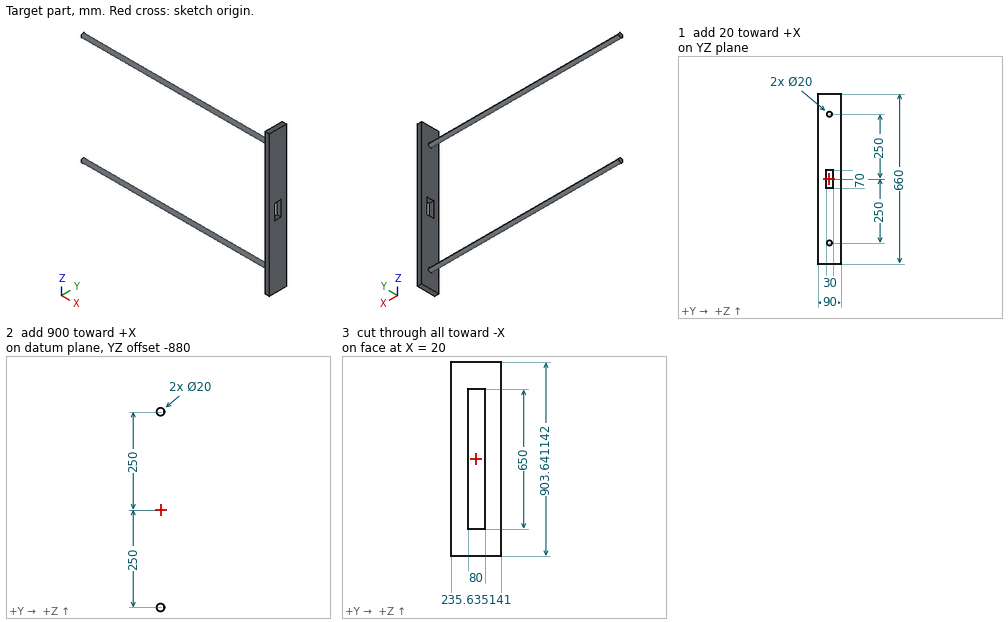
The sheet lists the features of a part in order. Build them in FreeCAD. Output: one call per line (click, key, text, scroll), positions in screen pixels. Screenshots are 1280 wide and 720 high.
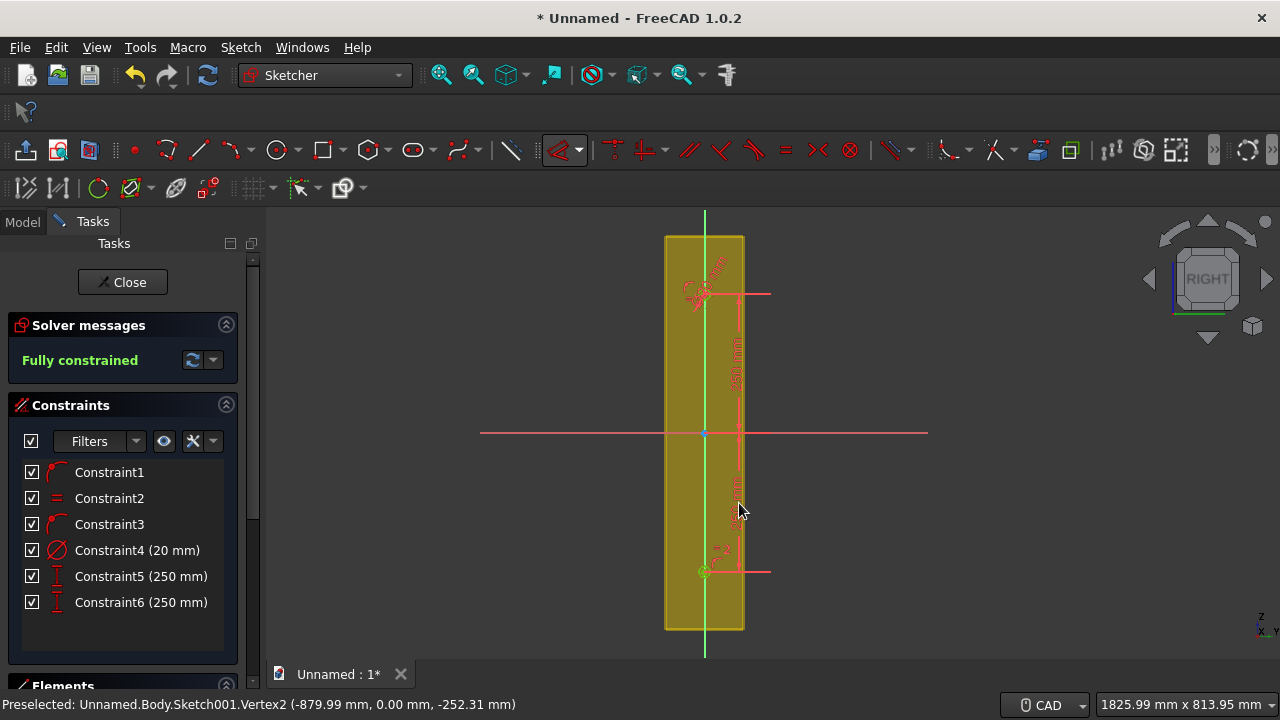
click(123, 282)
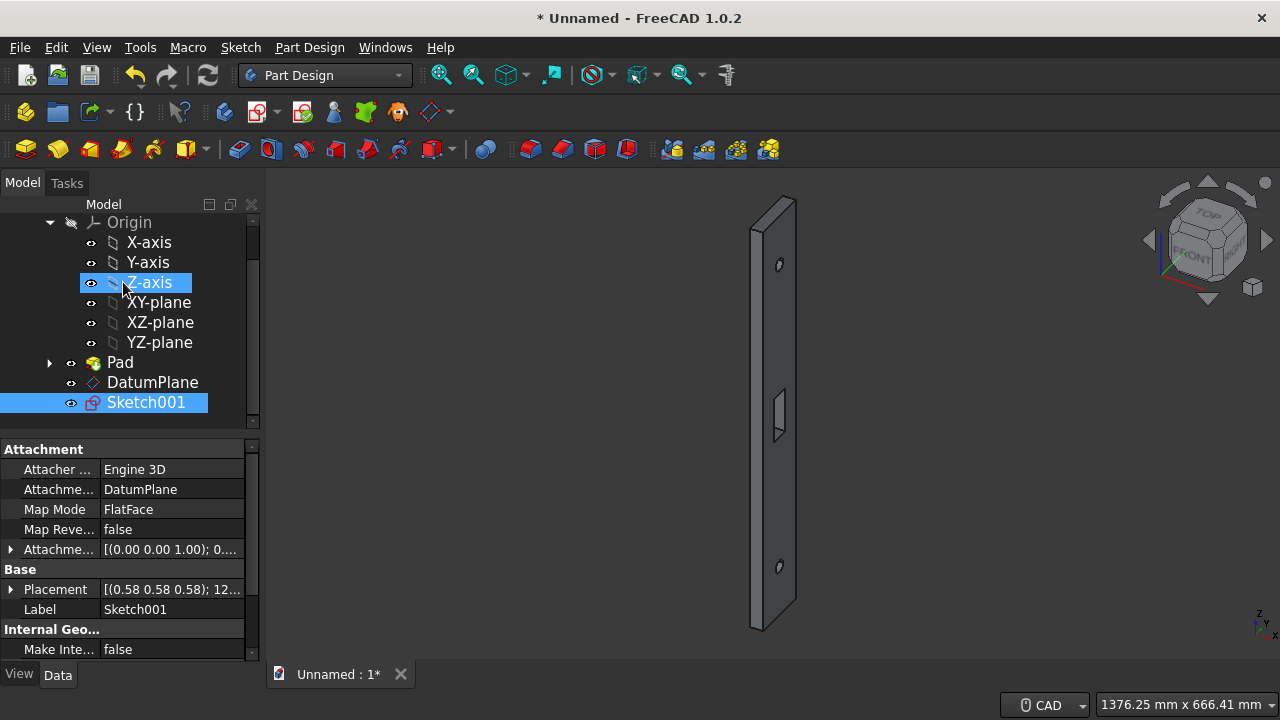
click(26, 150)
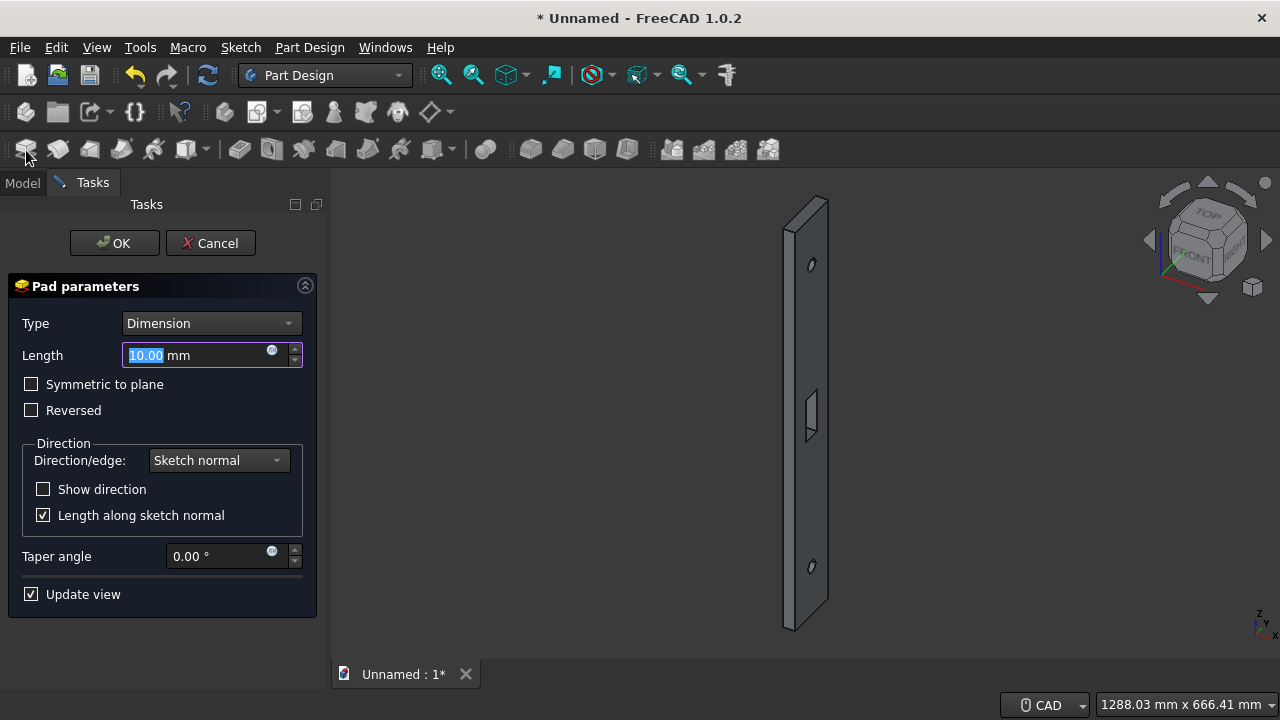
text(900)
key(Tab)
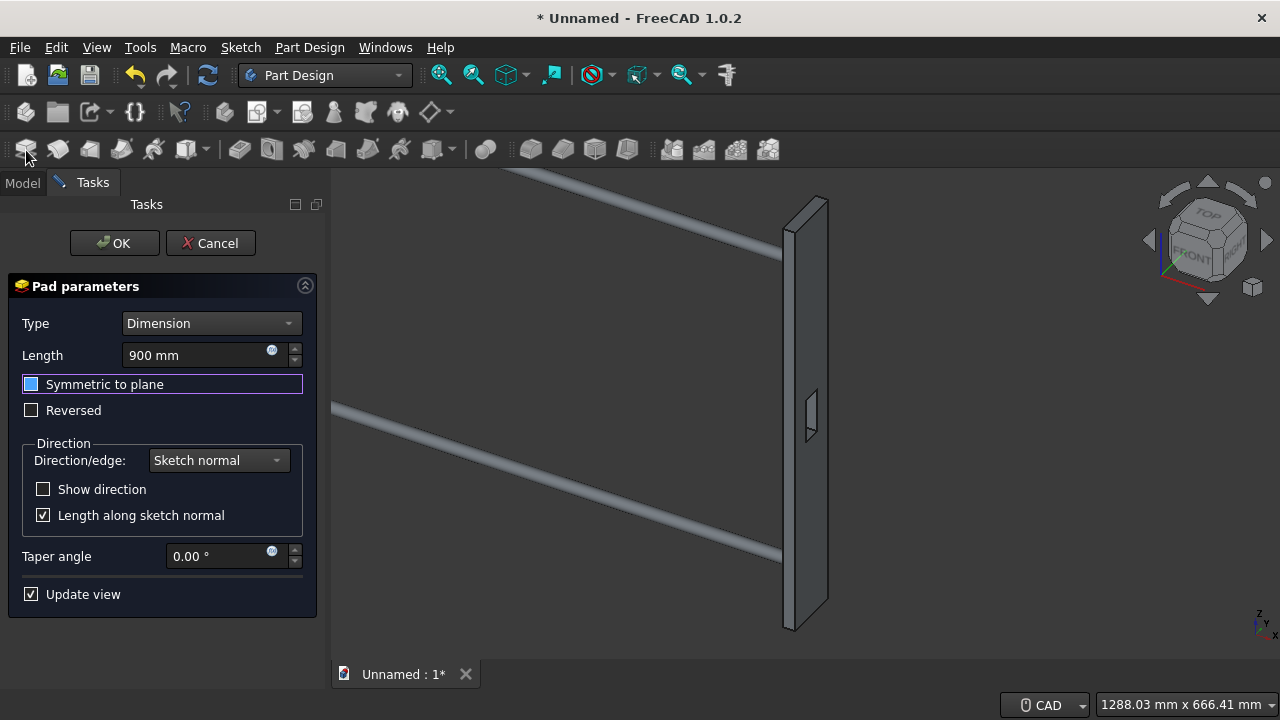
click(115, 243)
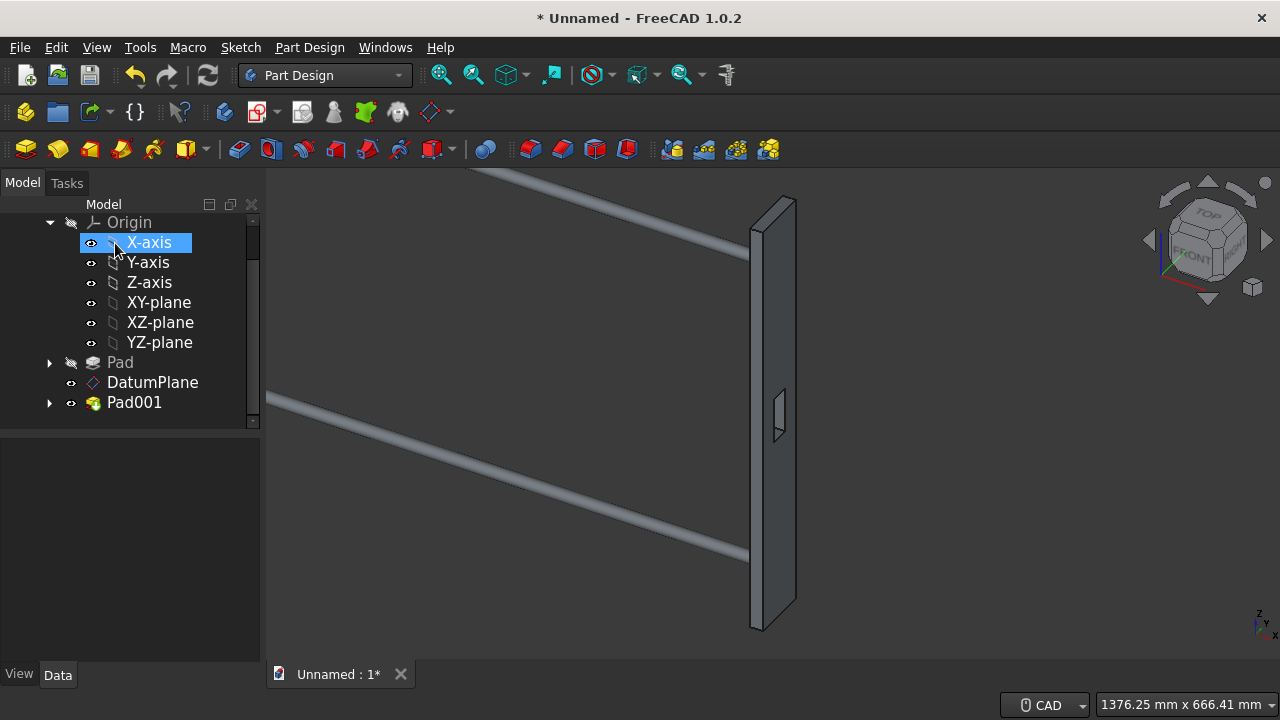
click(116, 383)
key(space)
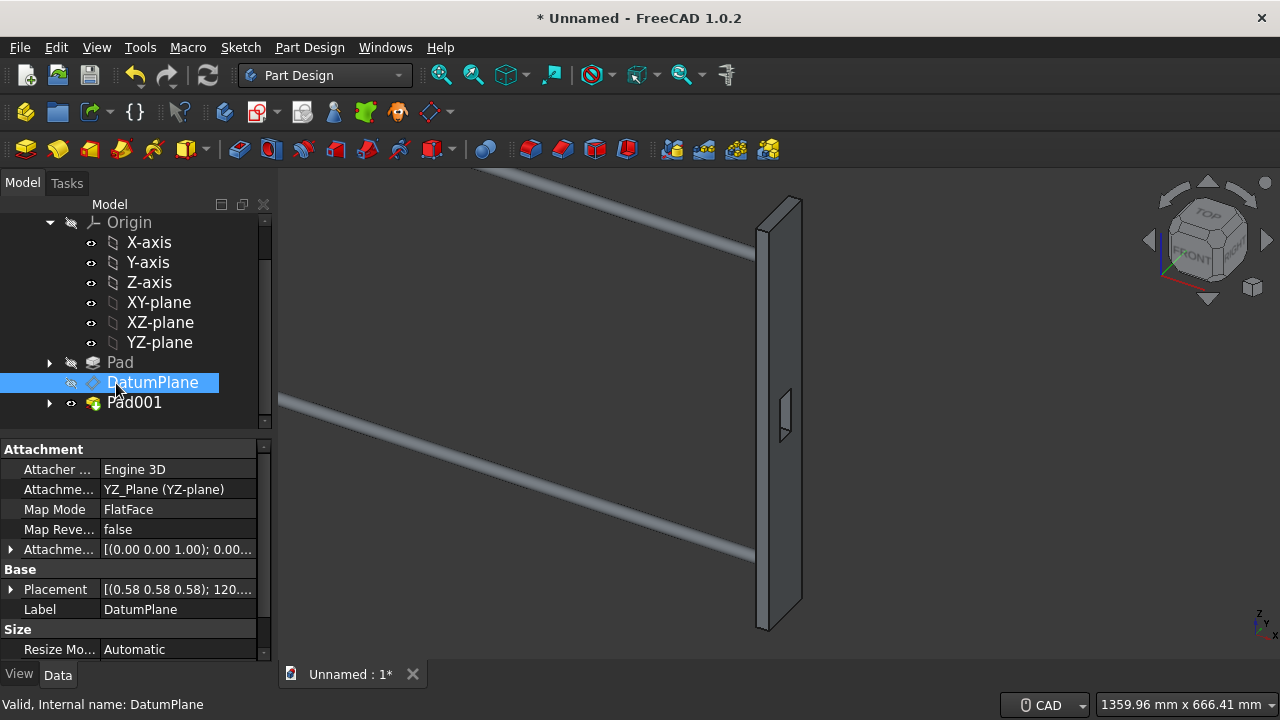
key(v)
key(f)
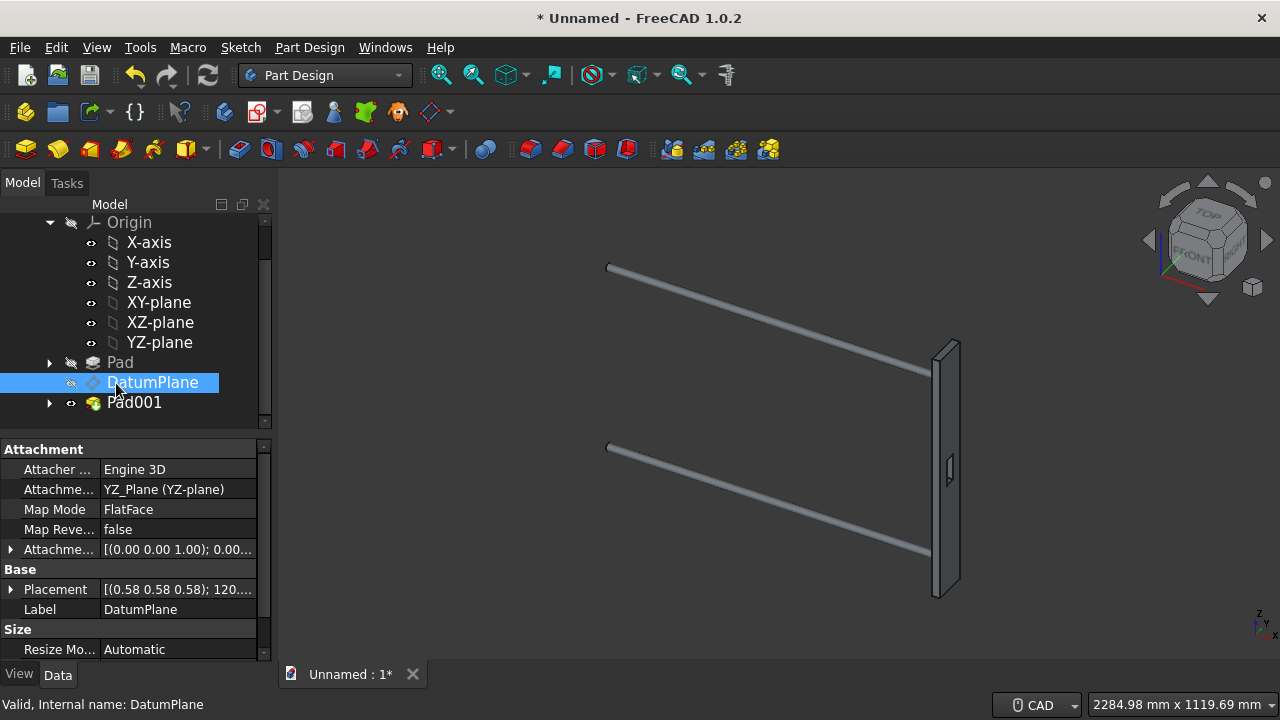
click(950, 435)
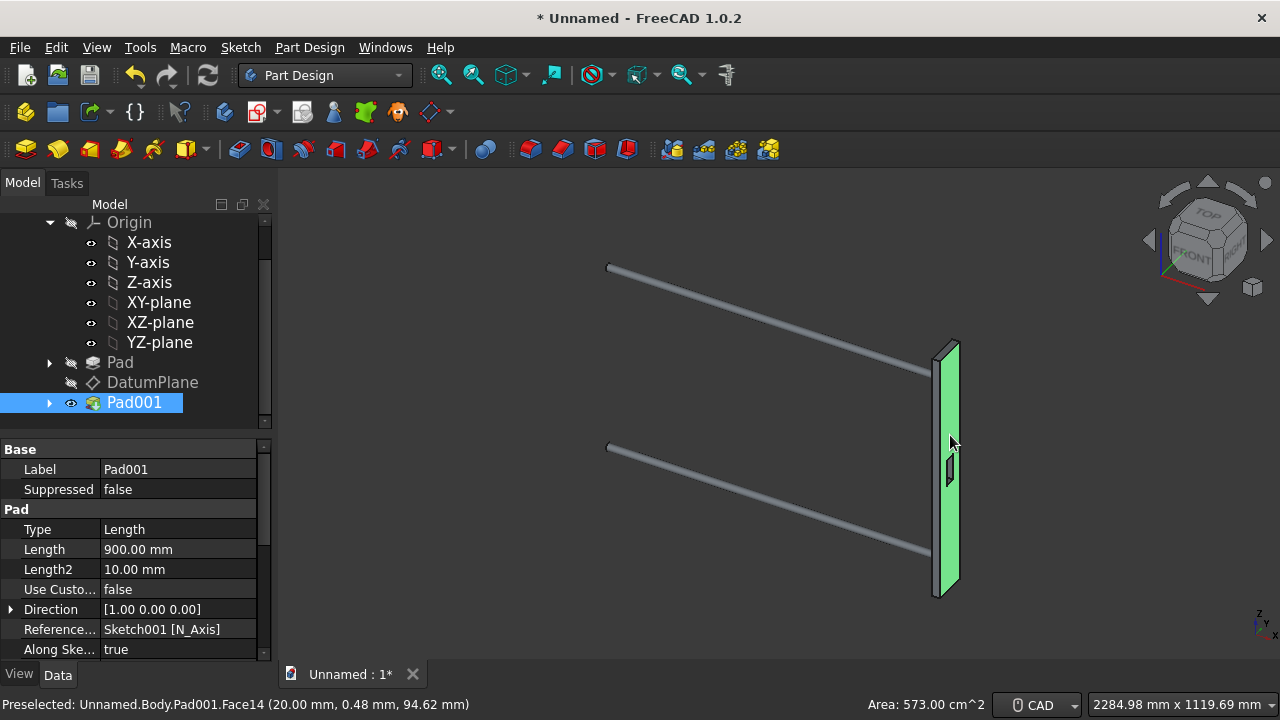
click(258, 112)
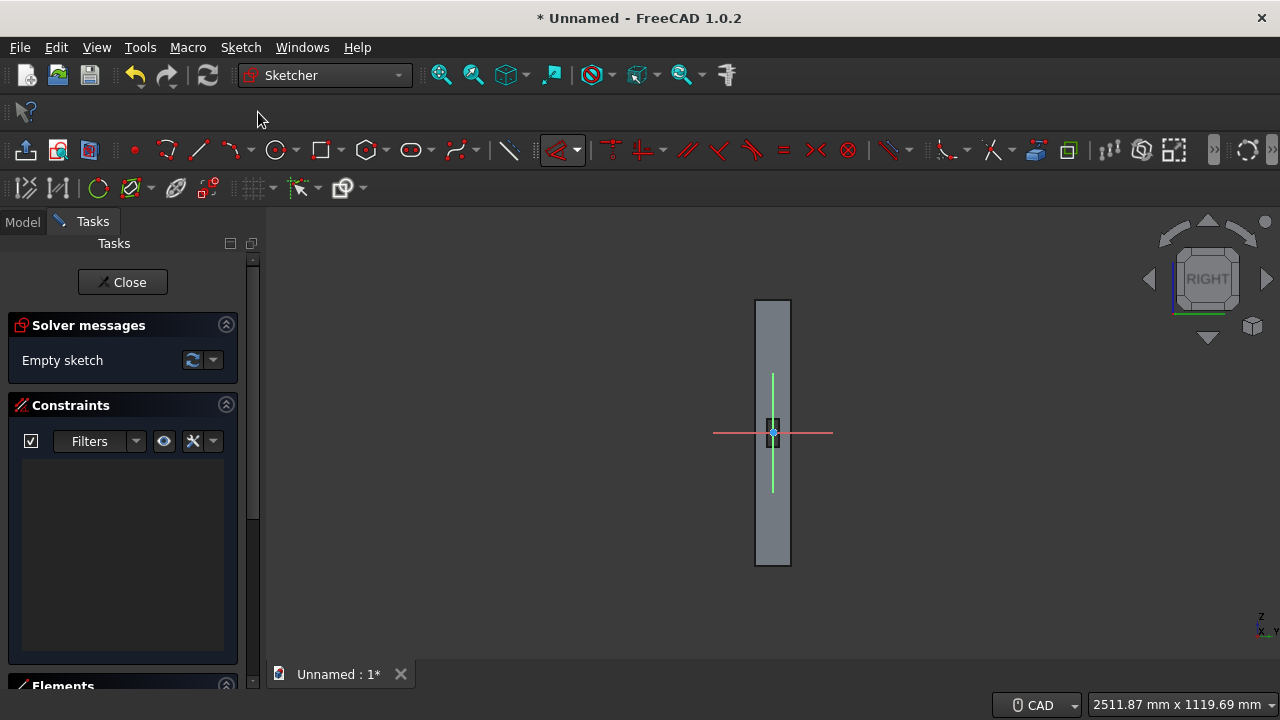
scroll(395, 433, down, 1)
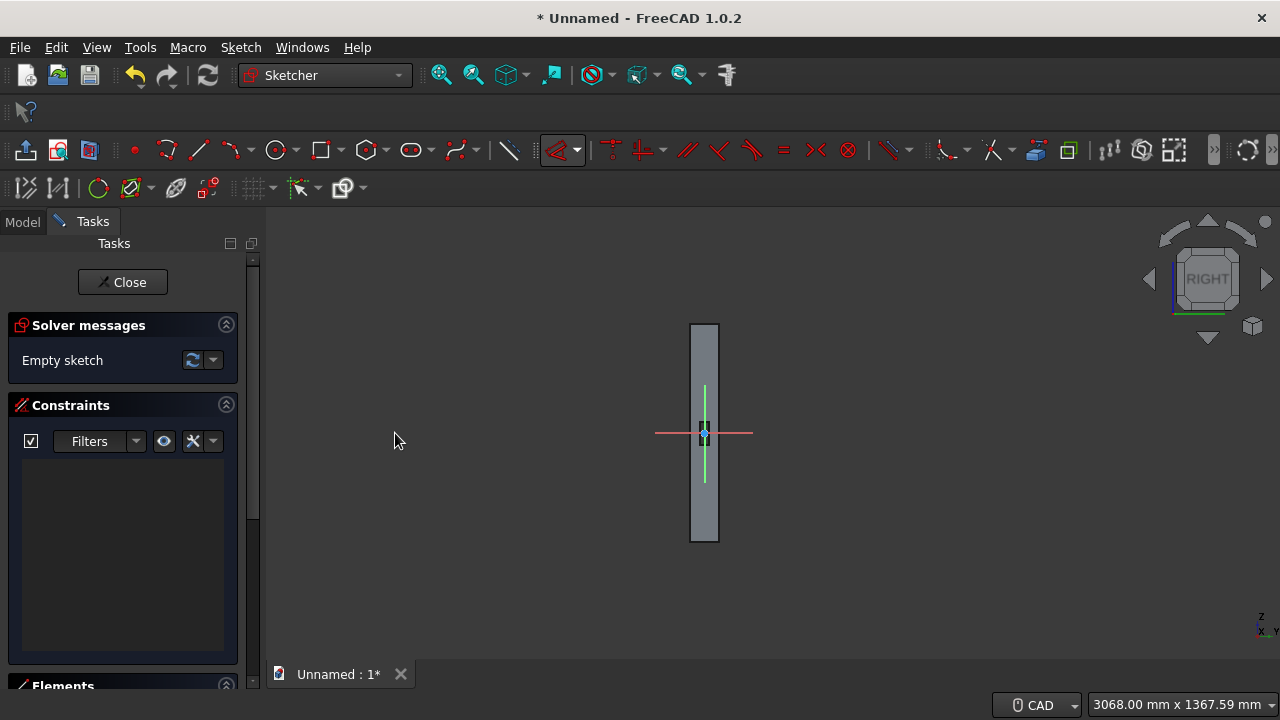
click(344, 150)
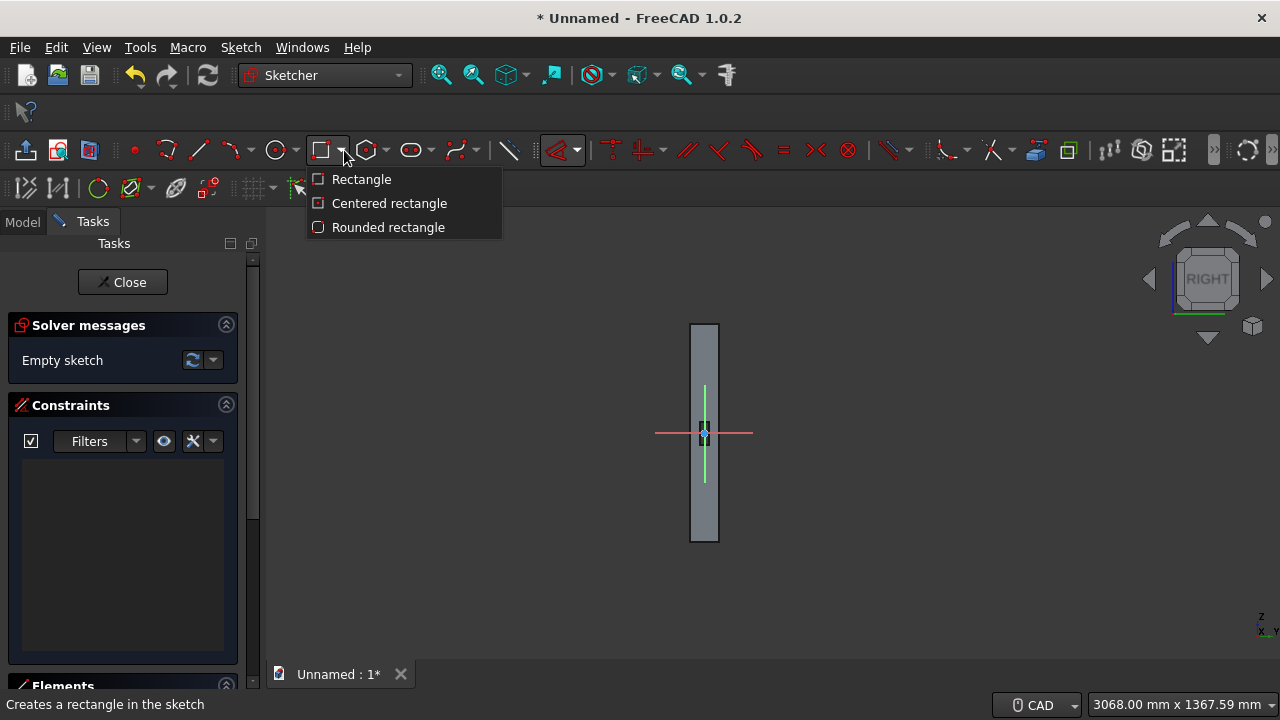
click(404, 203)